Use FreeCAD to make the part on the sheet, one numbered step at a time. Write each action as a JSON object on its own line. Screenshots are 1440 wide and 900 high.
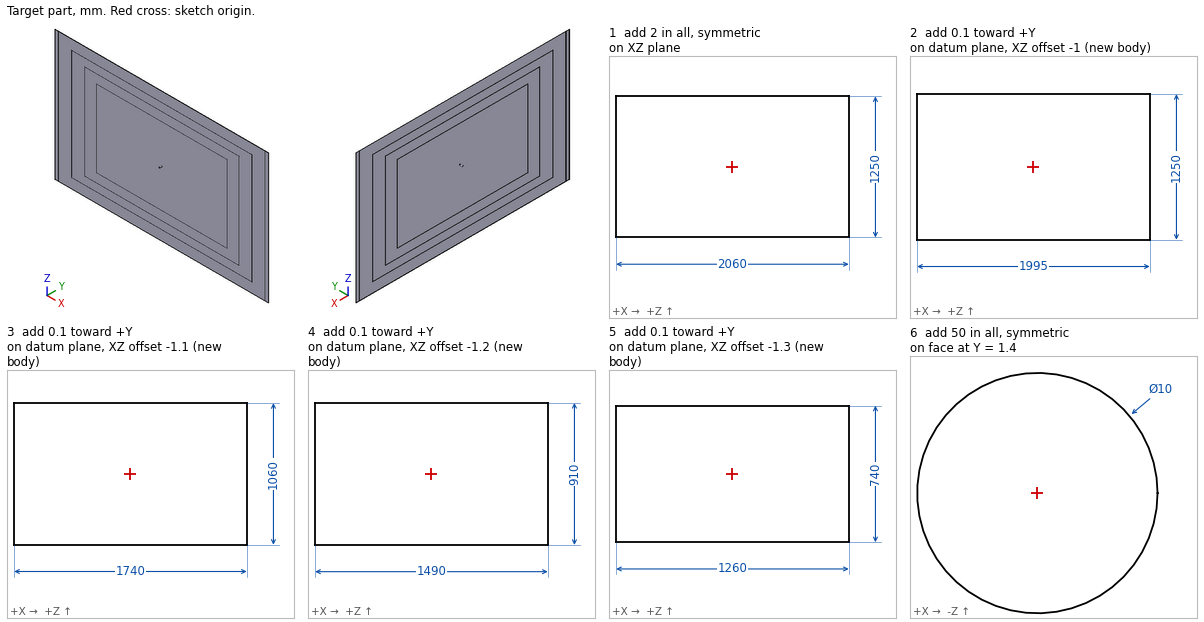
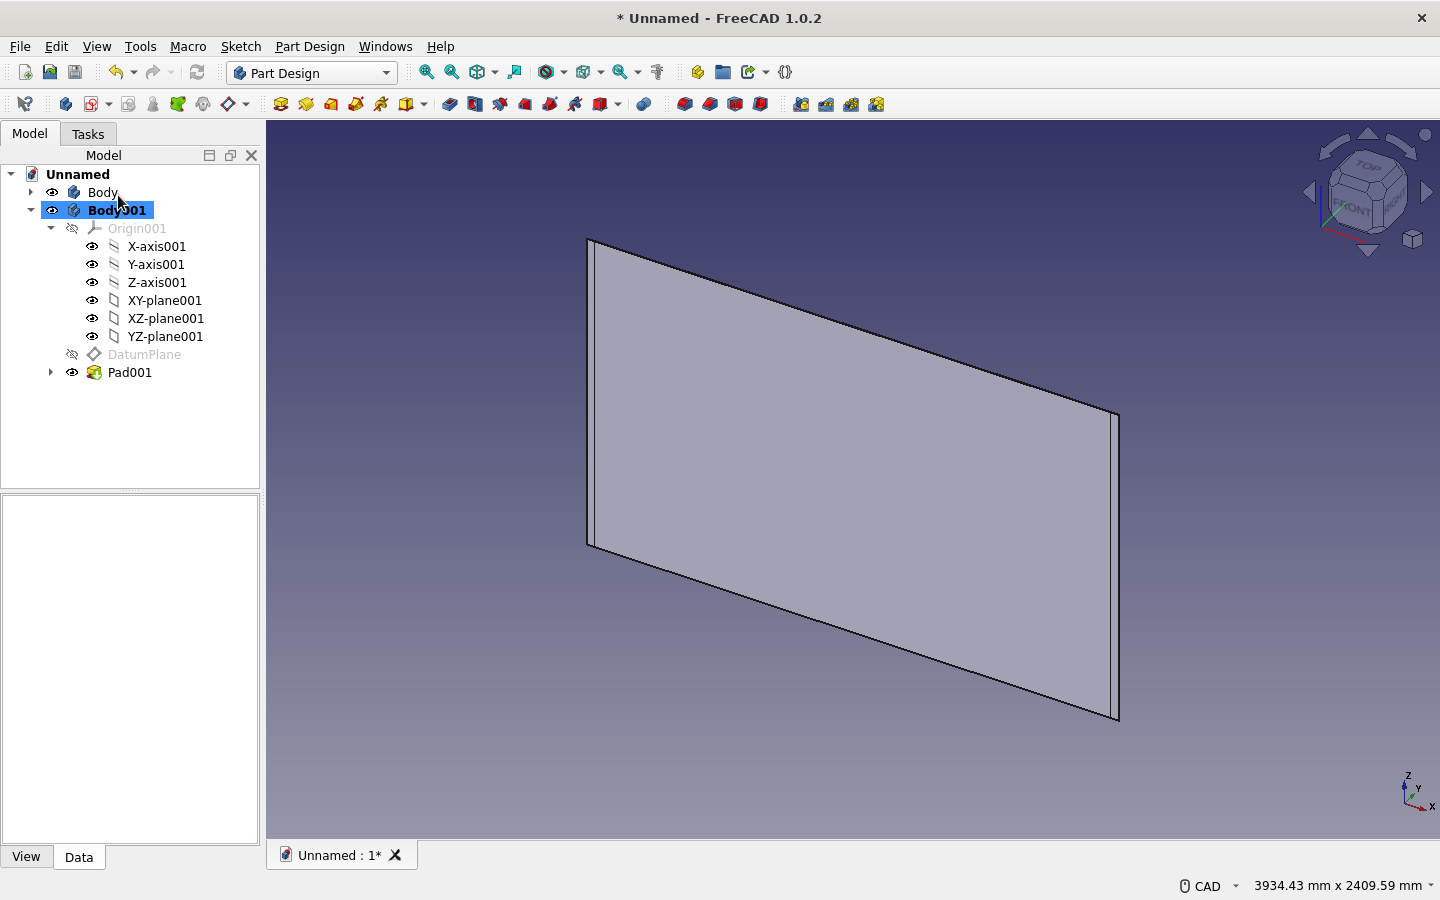
{"action": "left_click", "coordinate": [66, 104]}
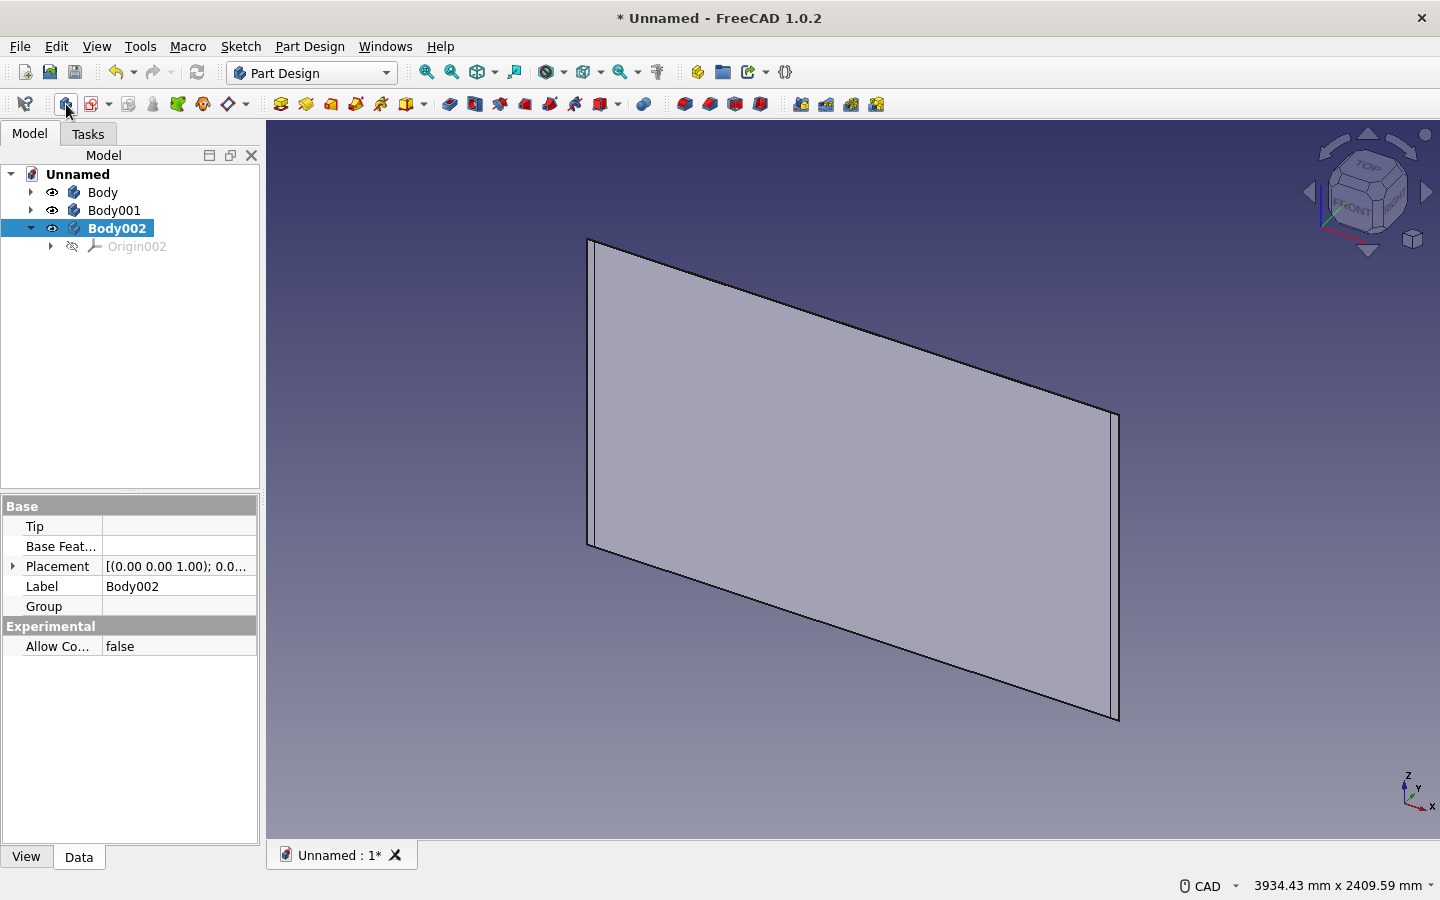
{"action": "left_click", "coordinate": [51, 246]}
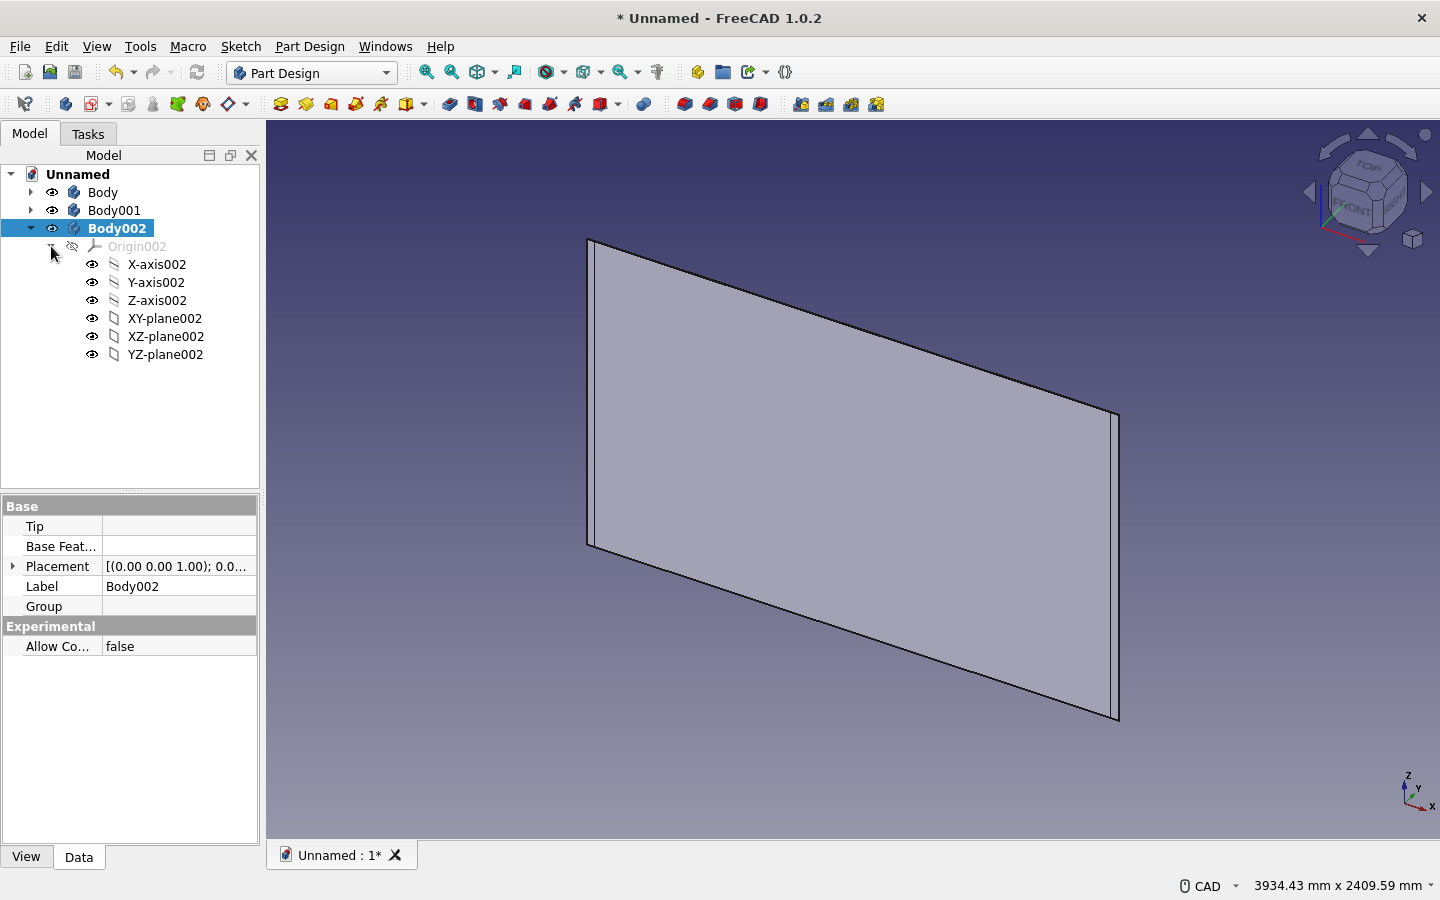
{"action": "left_click", "coordinate": [137, 336]}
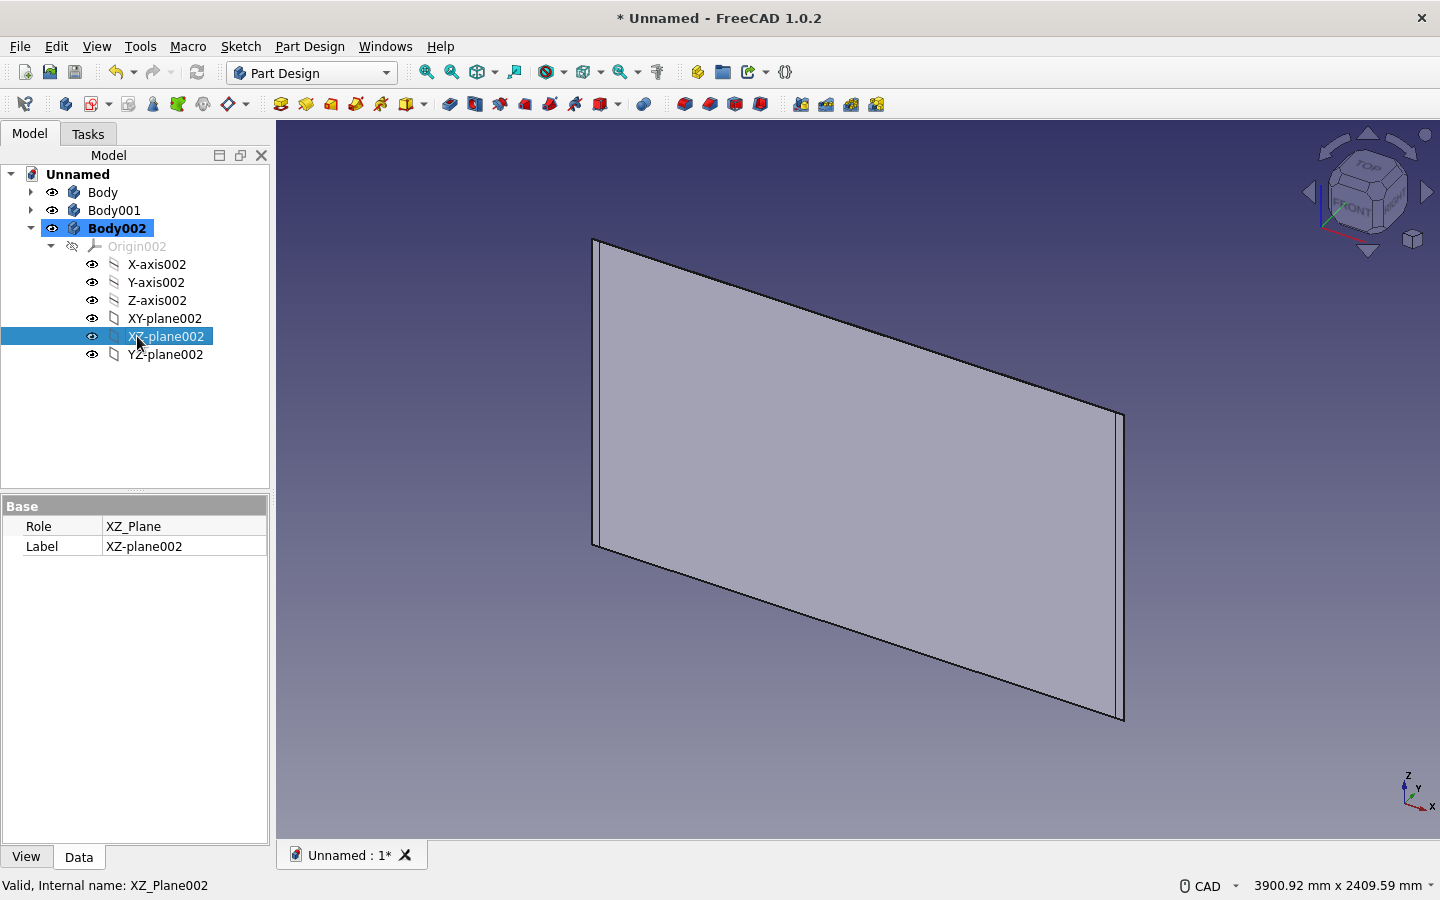
{"action": "left_click", "coordinate": [228, 104]}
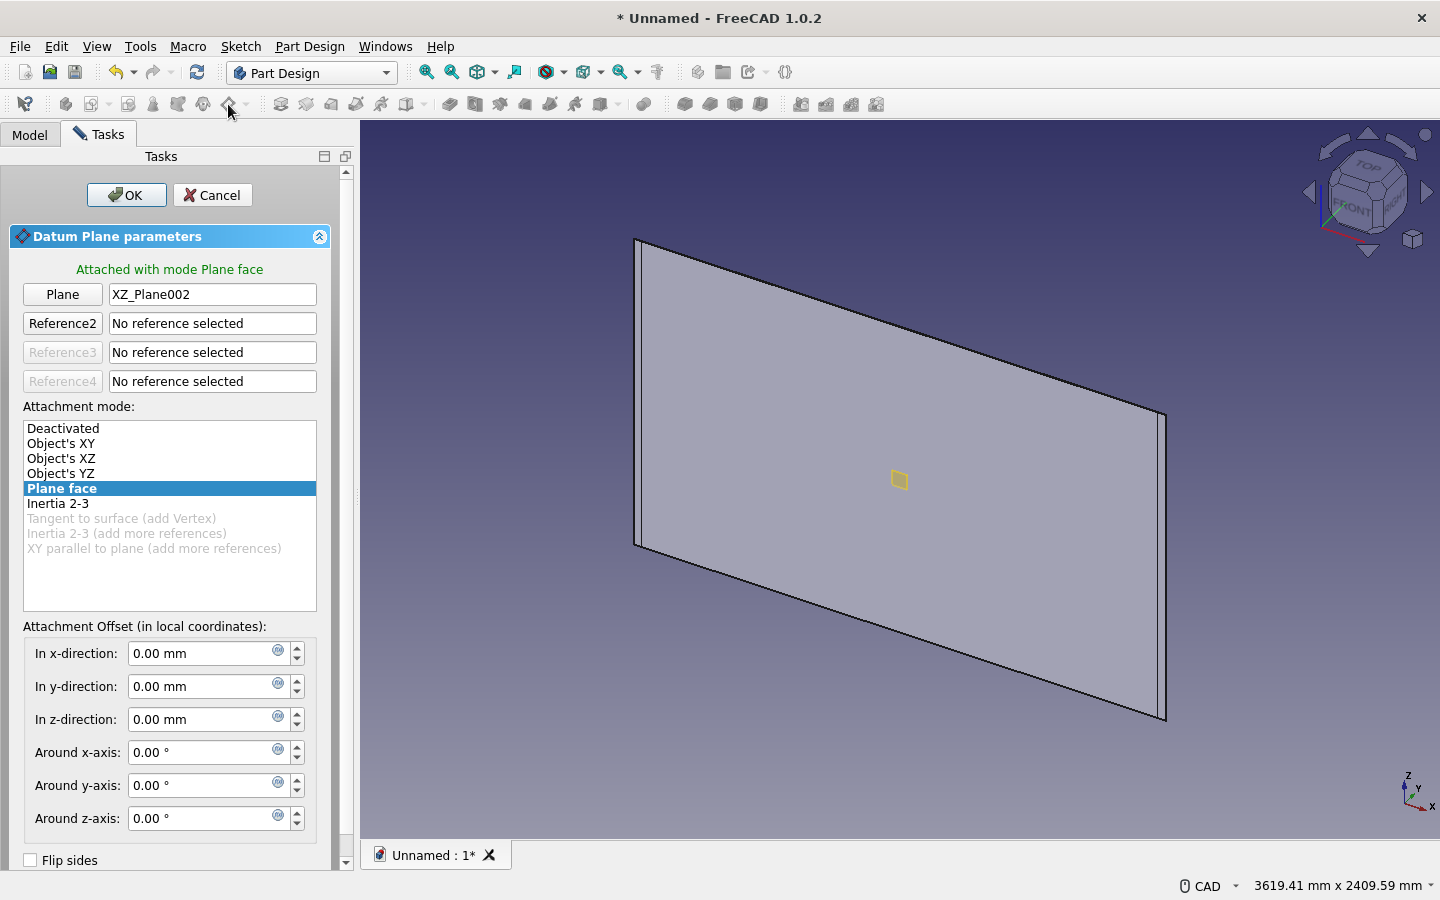
{"action": "triple_click", "coordinate": [210, 720]}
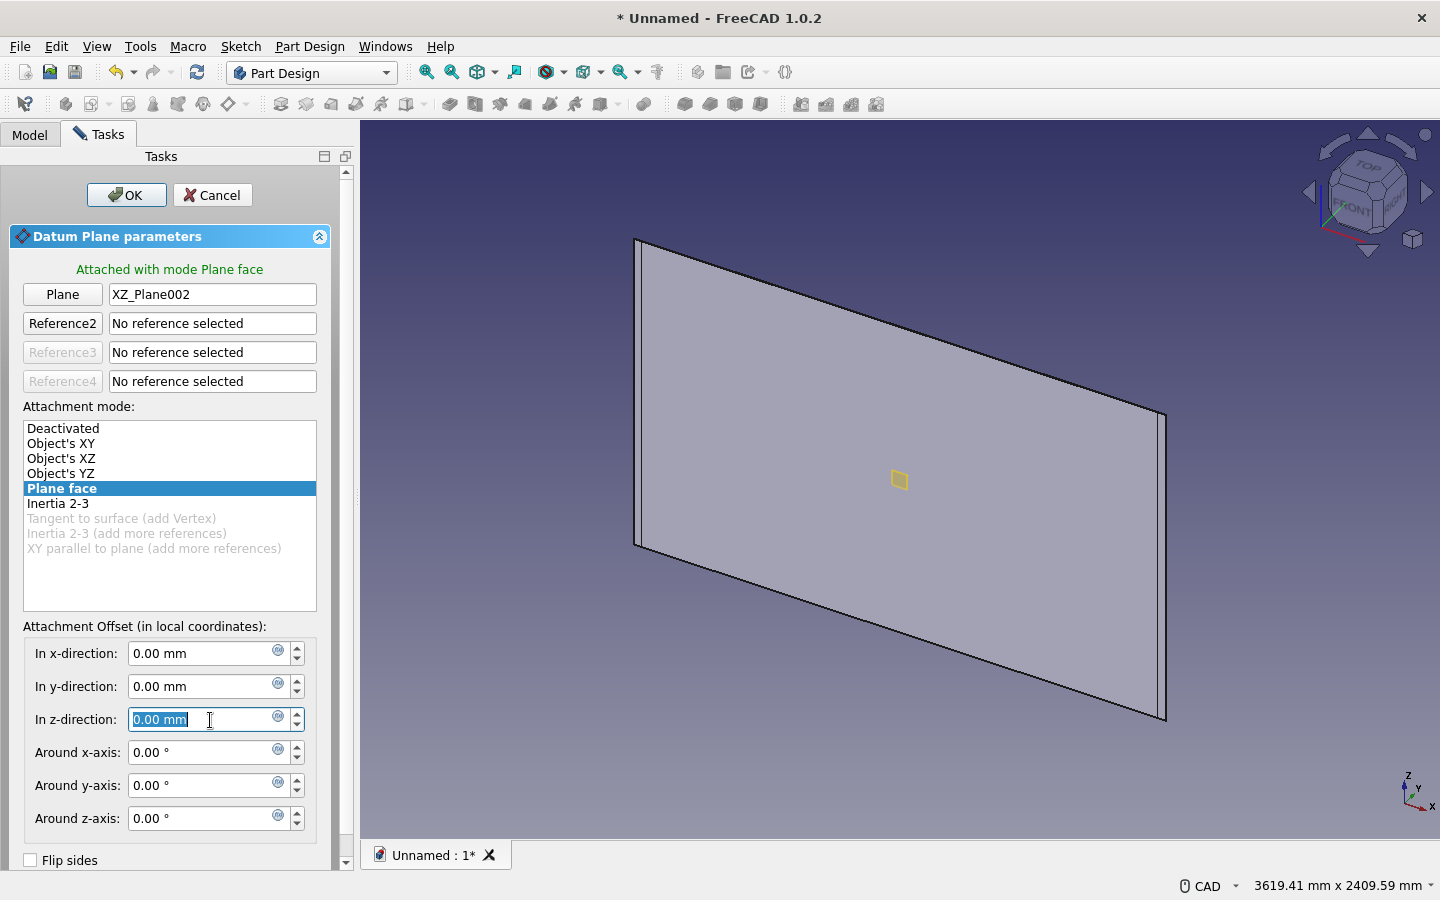
{"action": "type", "text": "-1.1"}
{"action": "key", "text": "Tab"}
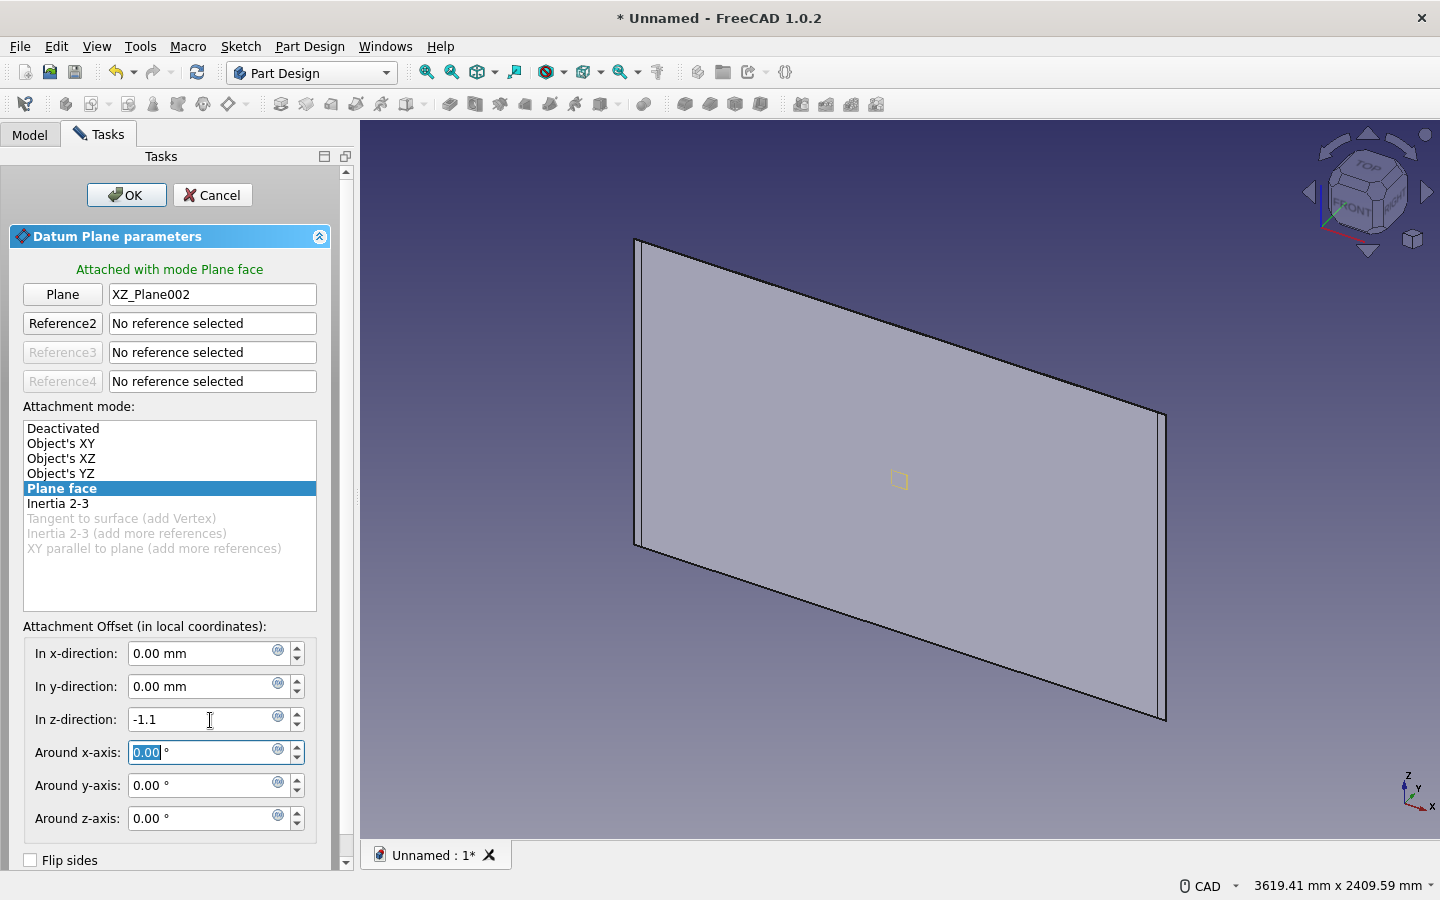
{"action": "left_click", "coordinate": [127, 195]}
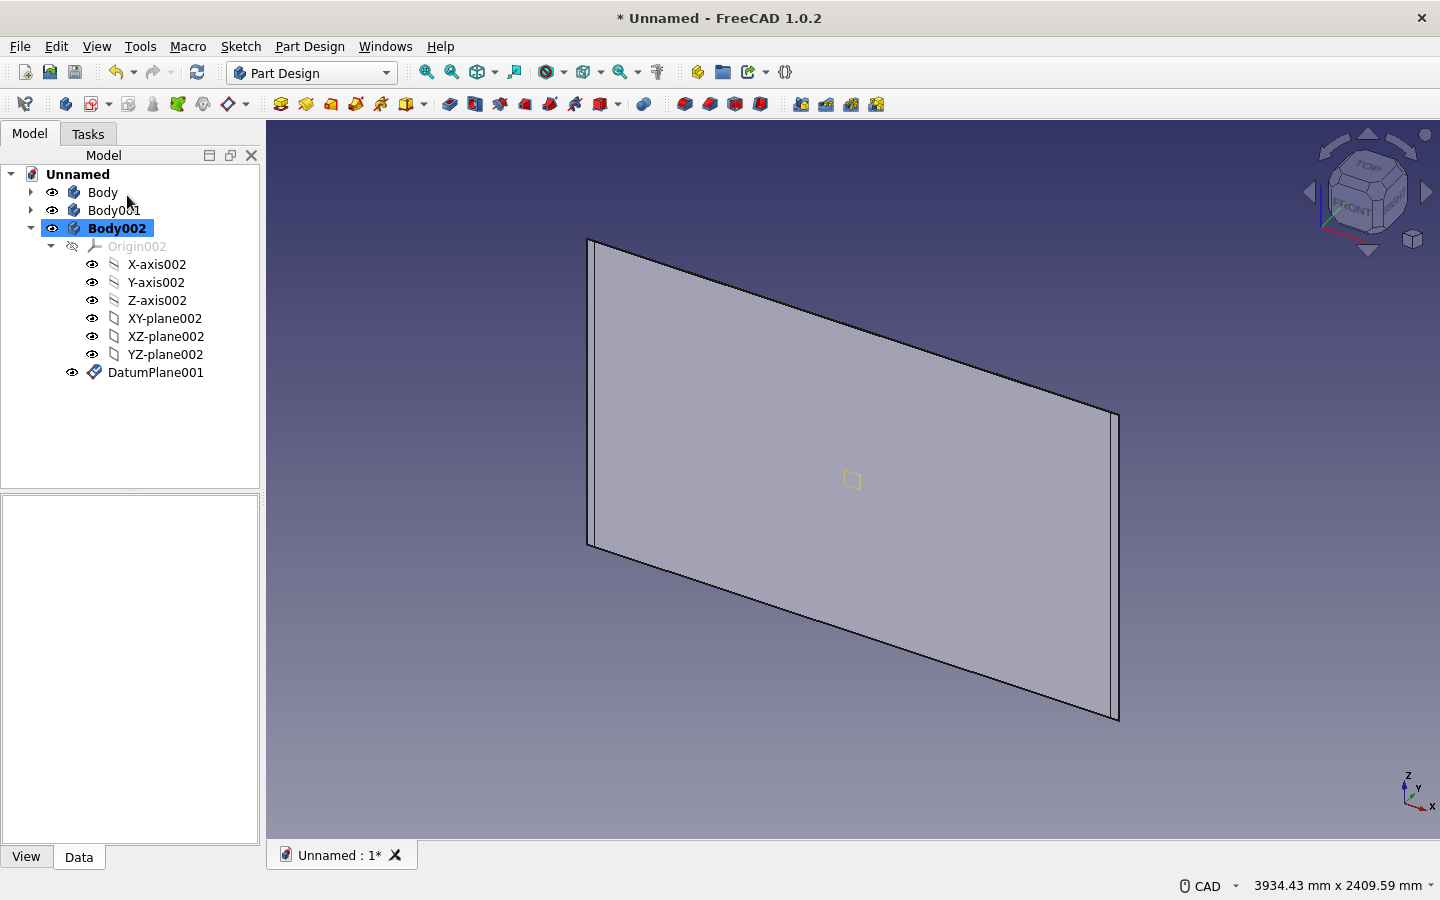
{"action": "left_click", "coordinate": [117, 372]}